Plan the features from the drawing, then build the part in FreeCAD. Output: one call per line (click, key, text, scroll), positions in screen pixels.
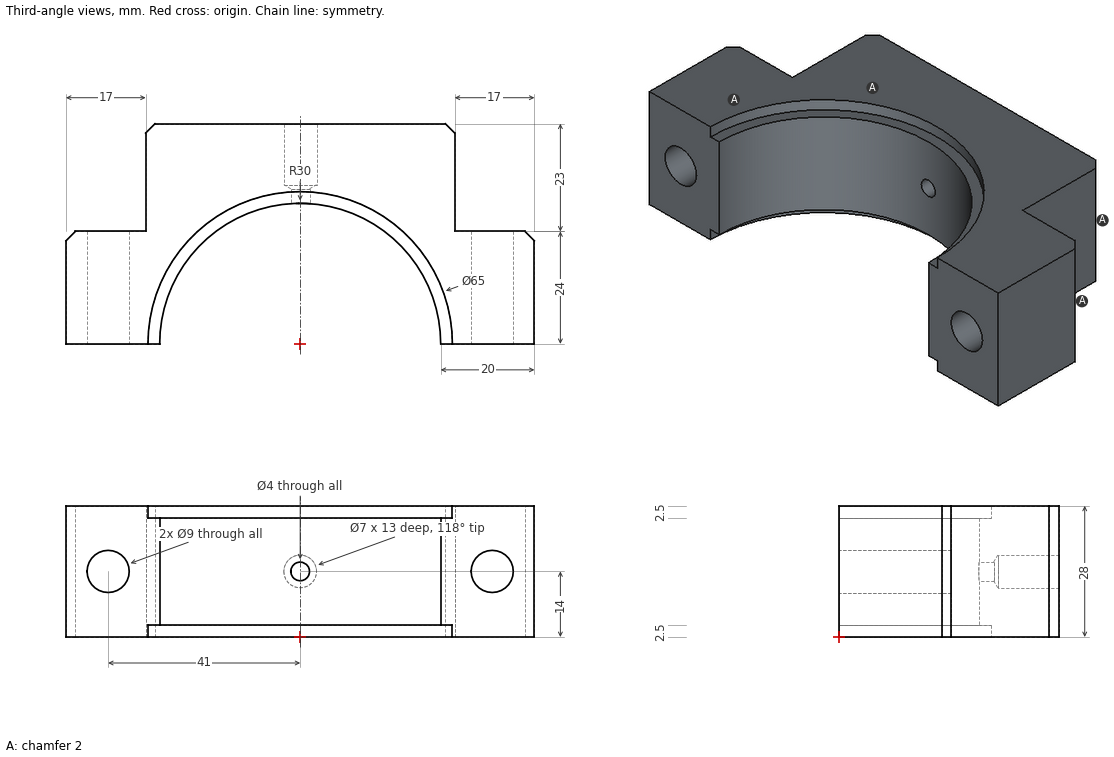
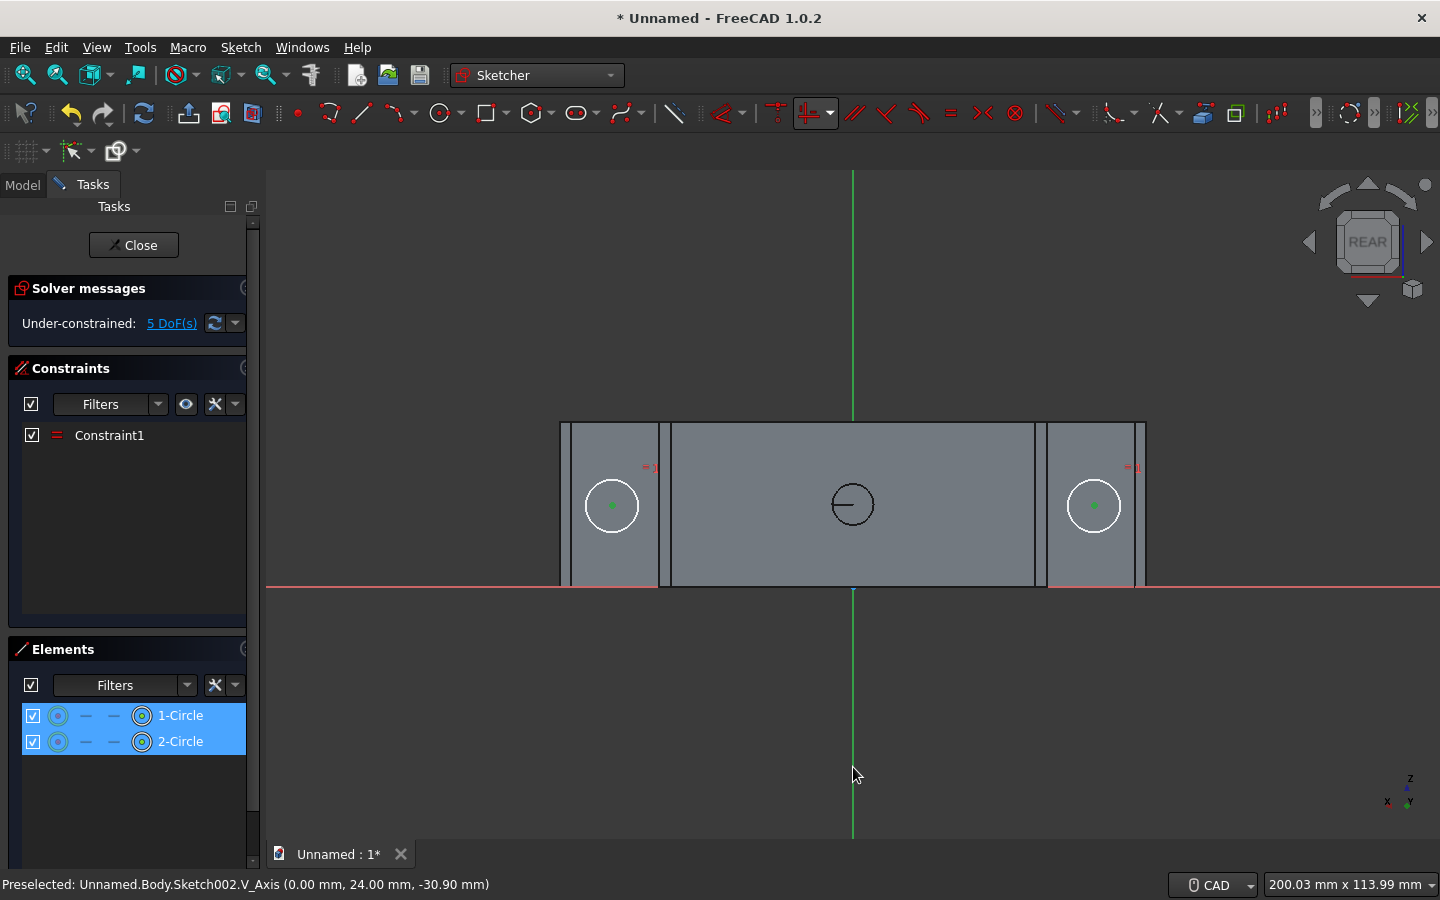
click(984, 114)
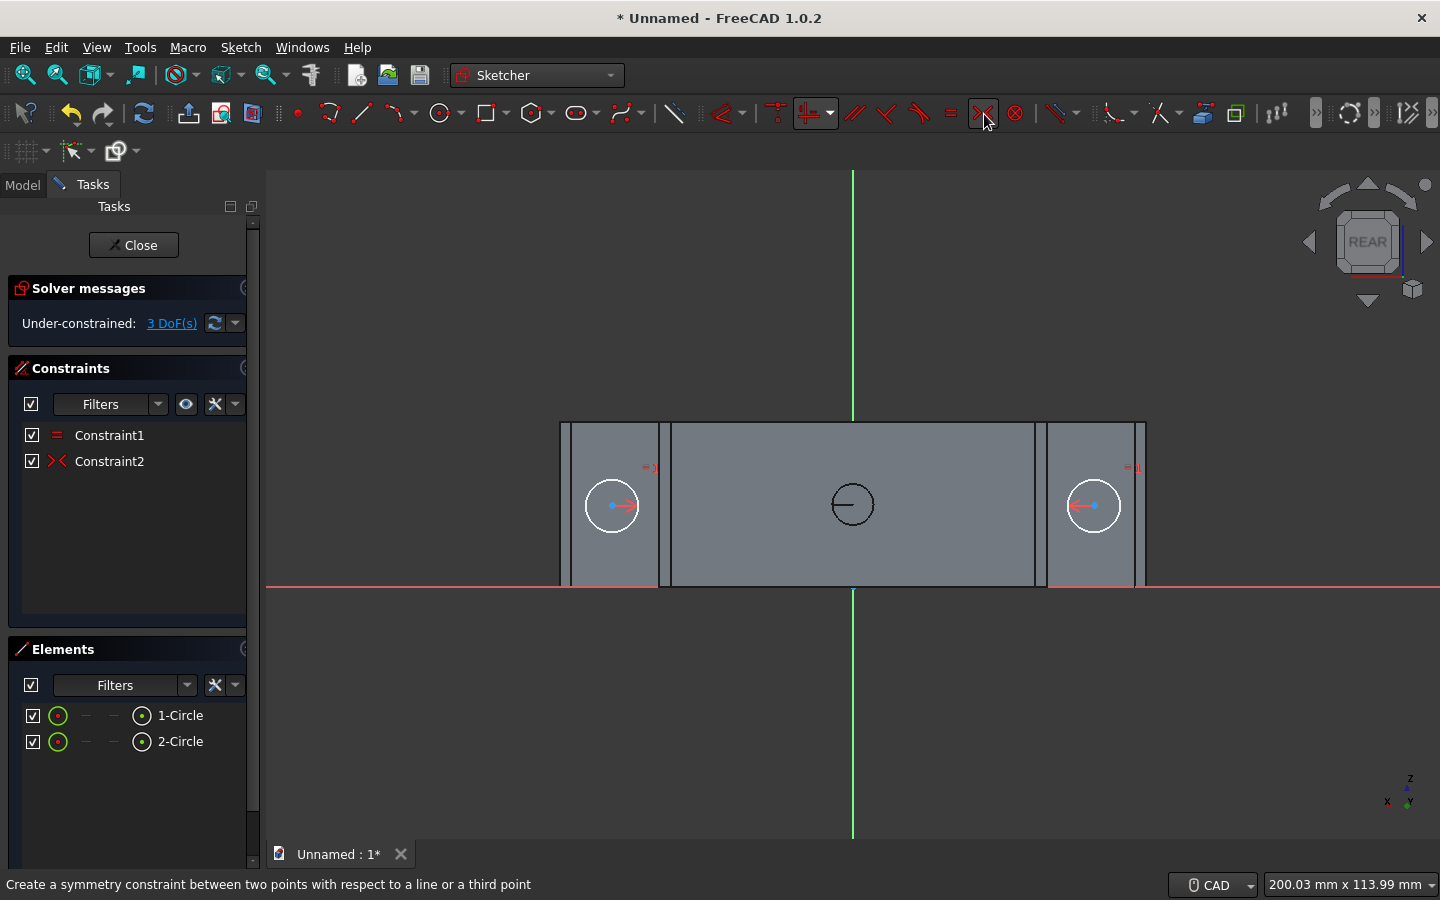
click(722, 114)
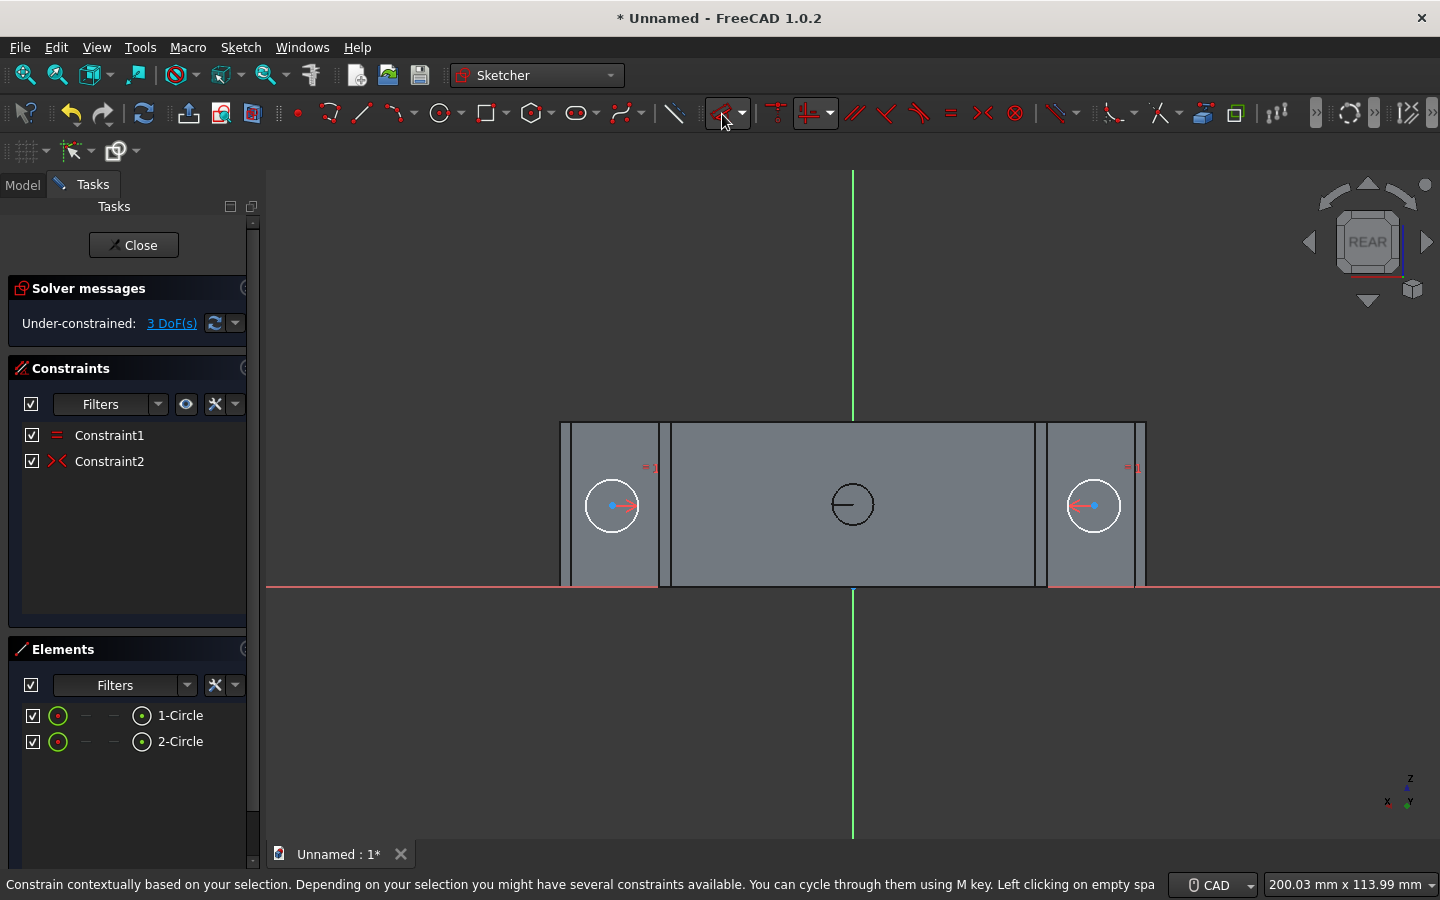
click(1112, 487)
click(1134, 464)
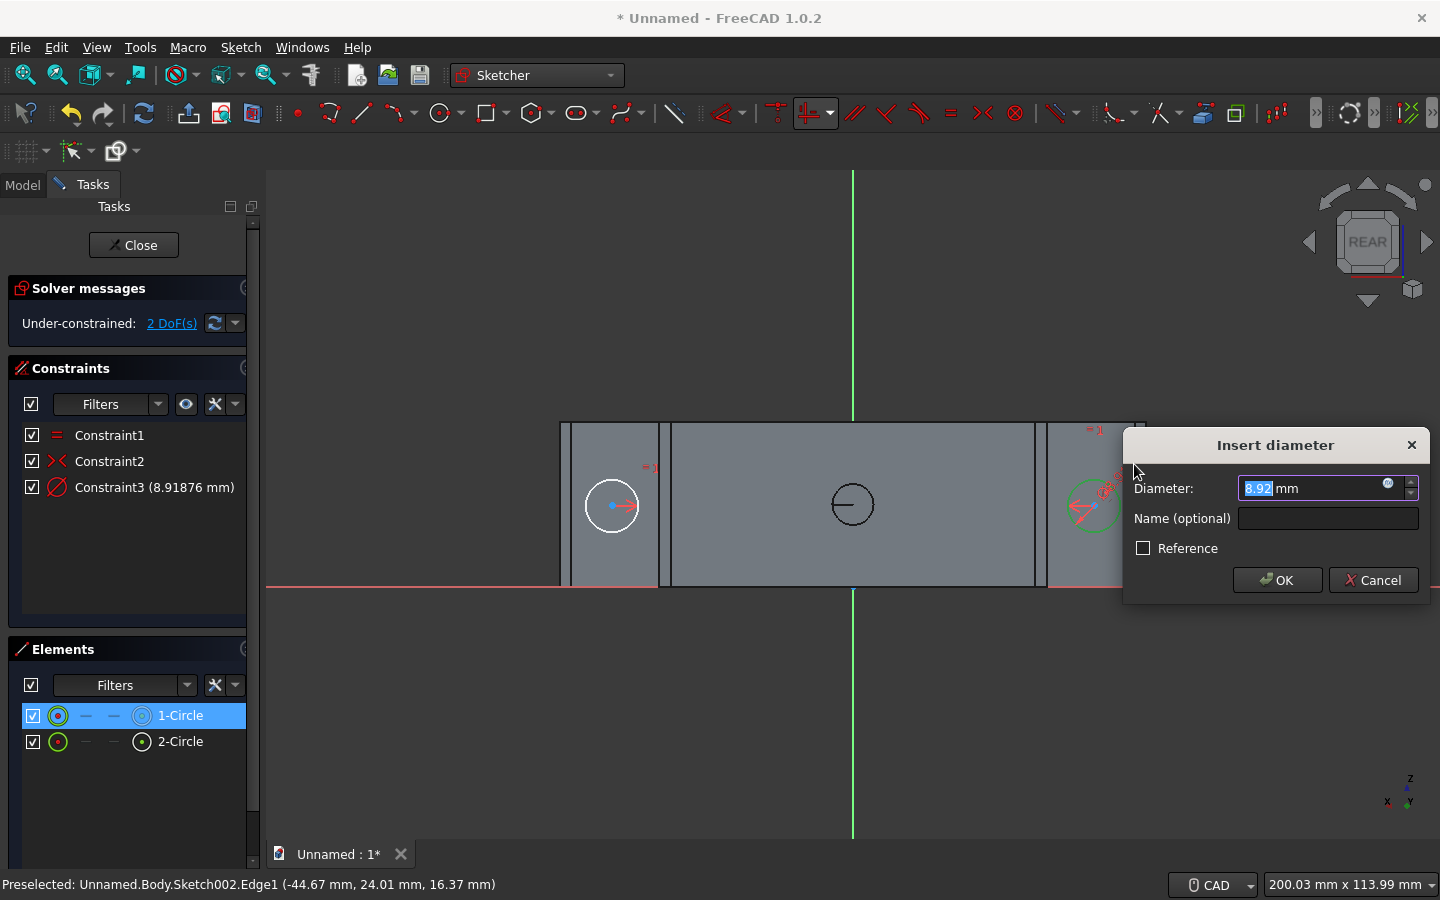
text(9)
key(Return)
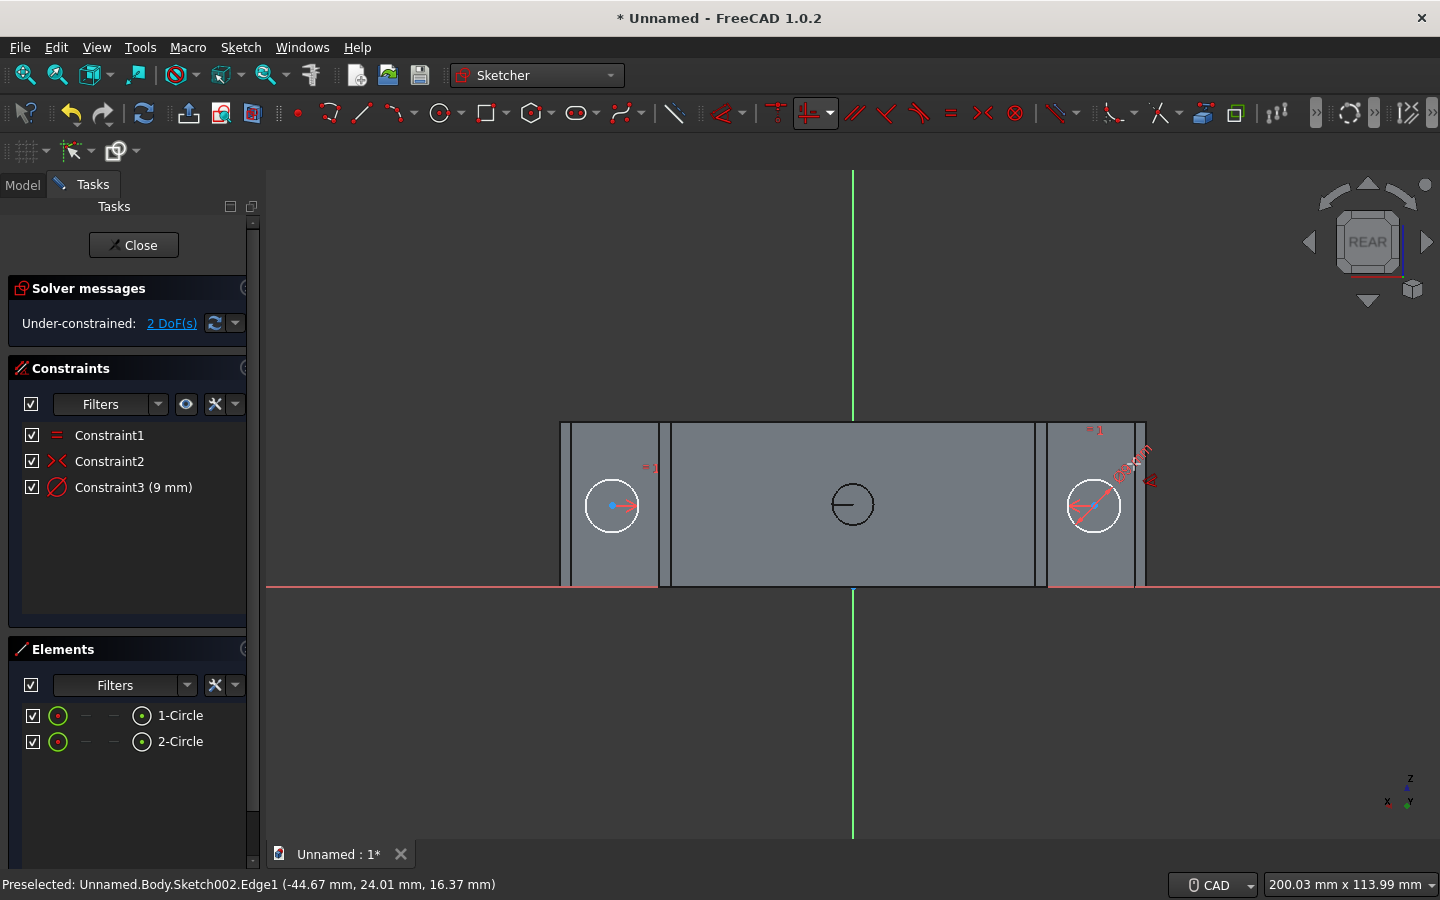
click(1094, 506)
click(974, 621)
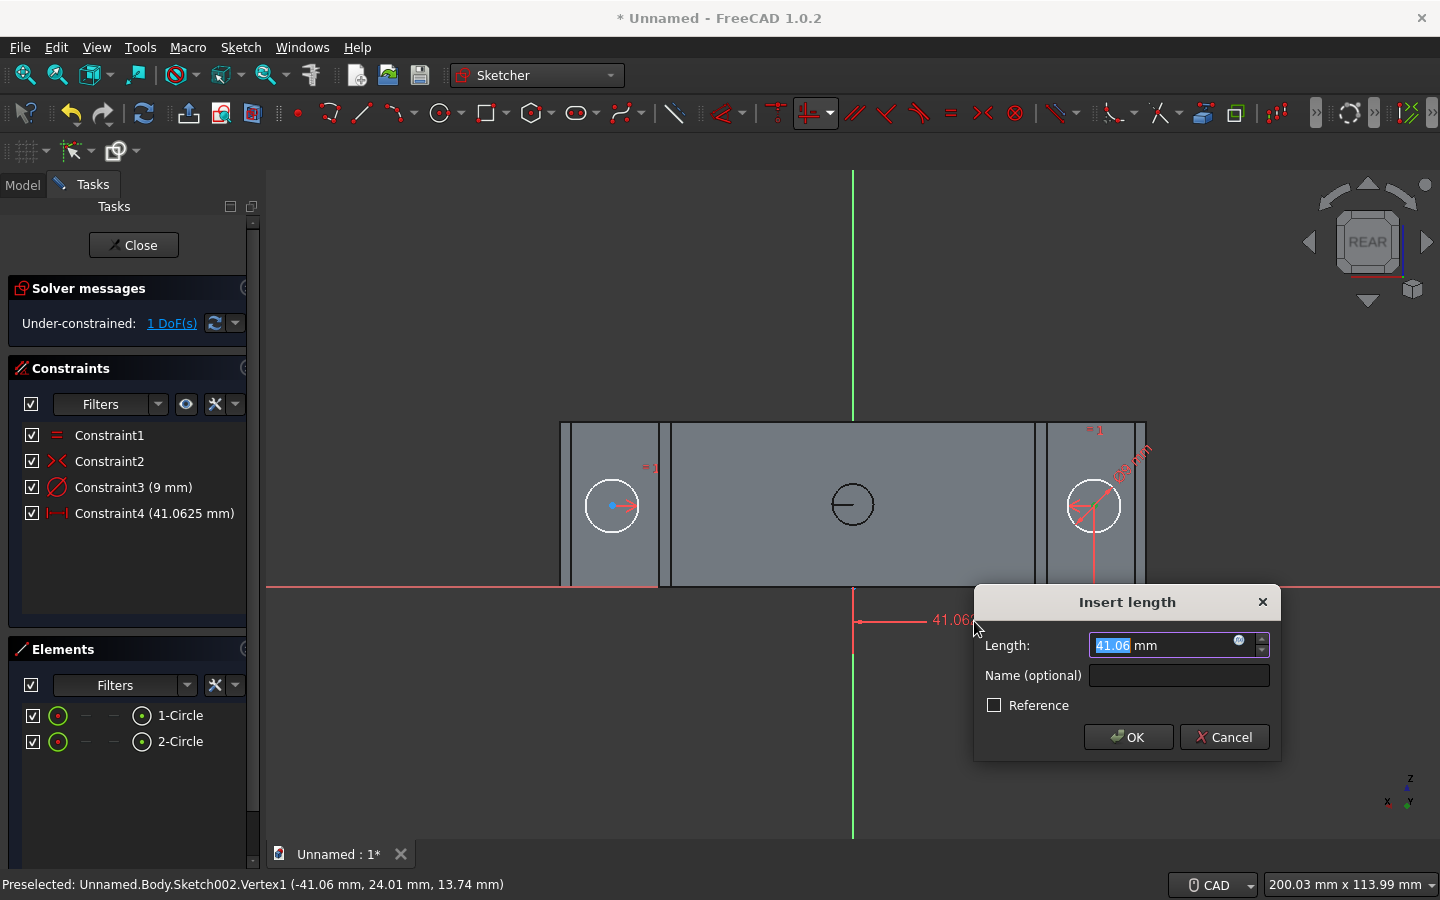
text(41)
key(Return)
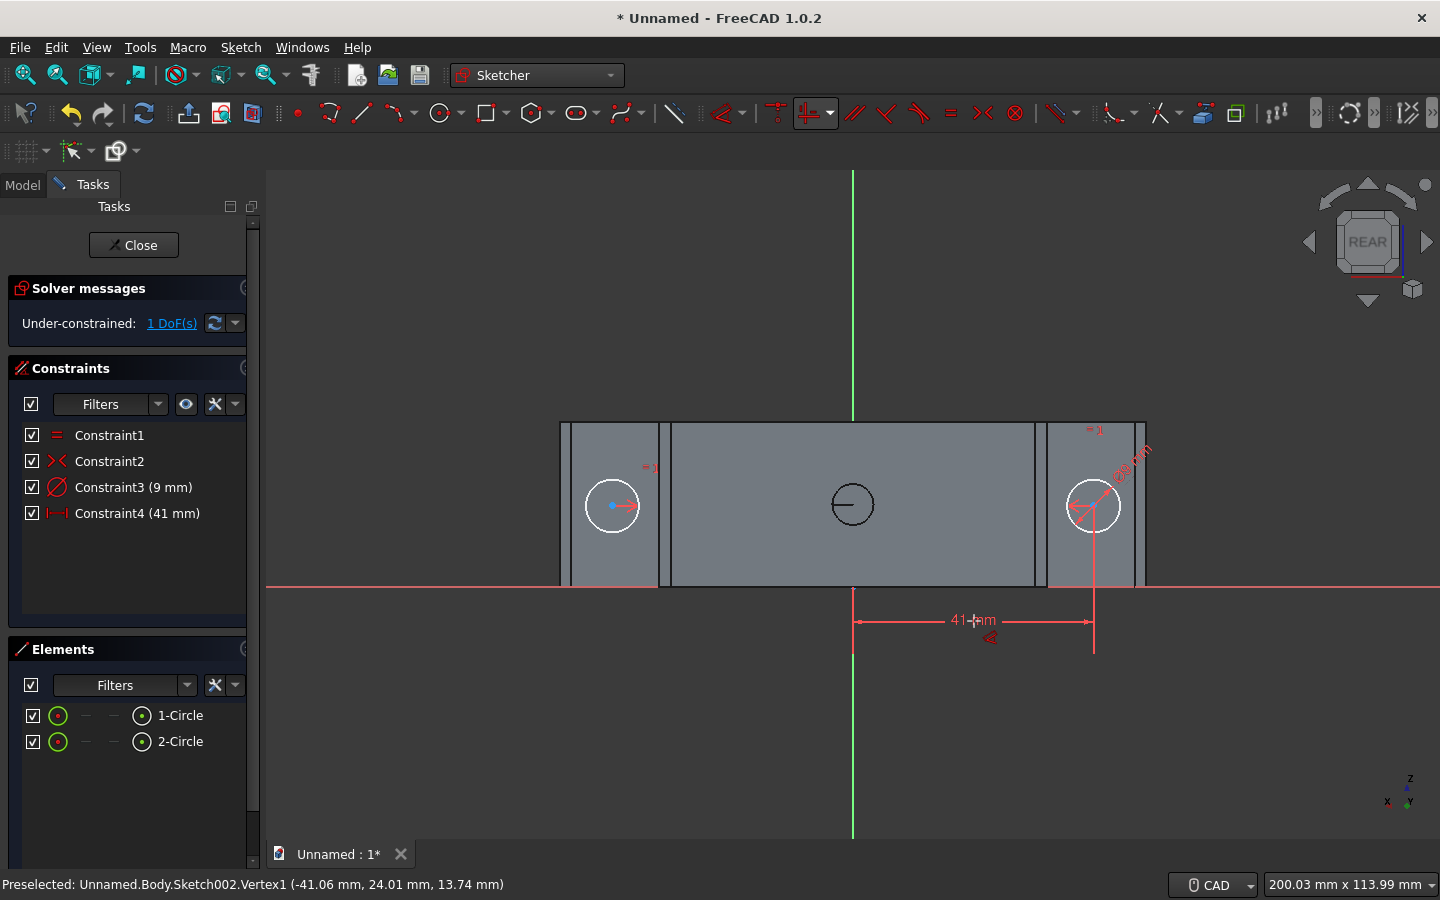
click(1094, 506)
click(1128, 546)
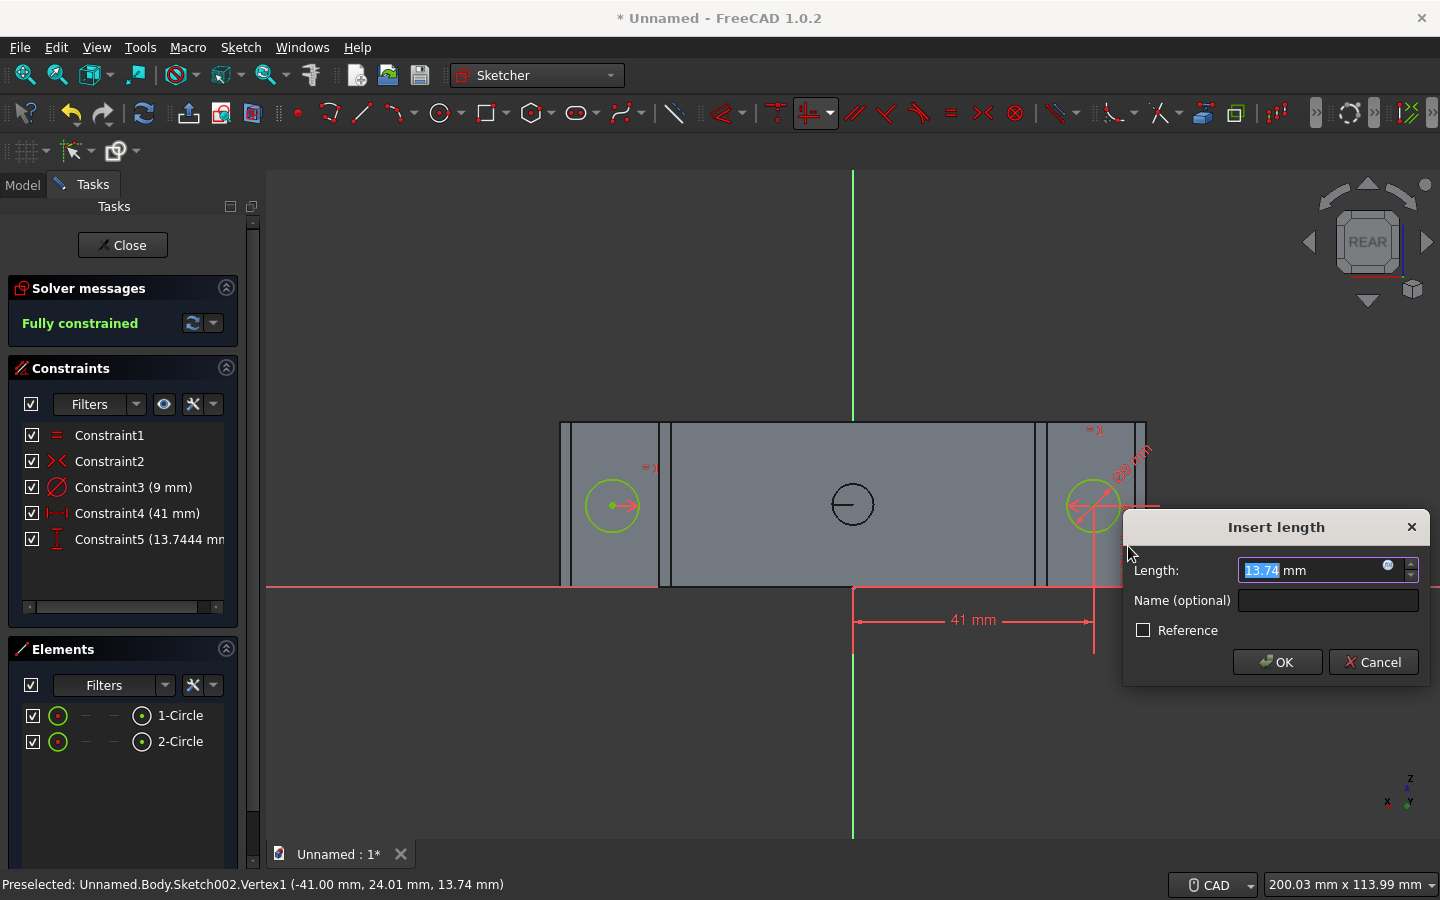
text(14)
key(Return)
key(Escape)